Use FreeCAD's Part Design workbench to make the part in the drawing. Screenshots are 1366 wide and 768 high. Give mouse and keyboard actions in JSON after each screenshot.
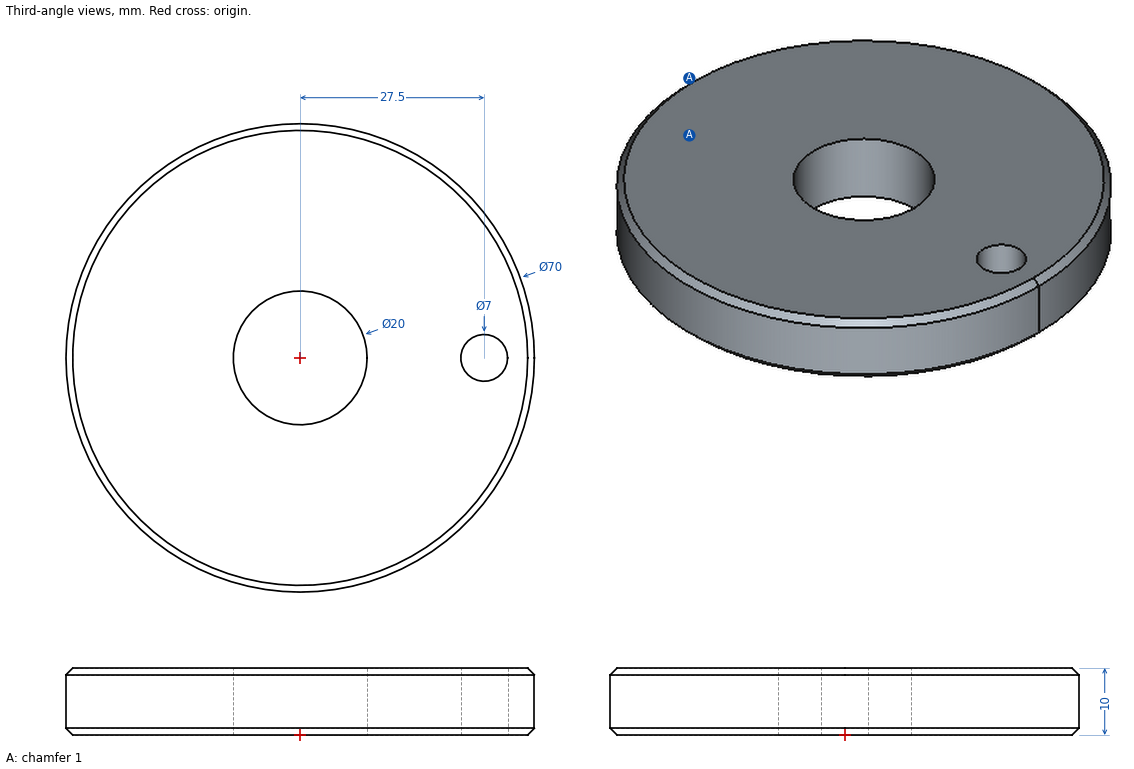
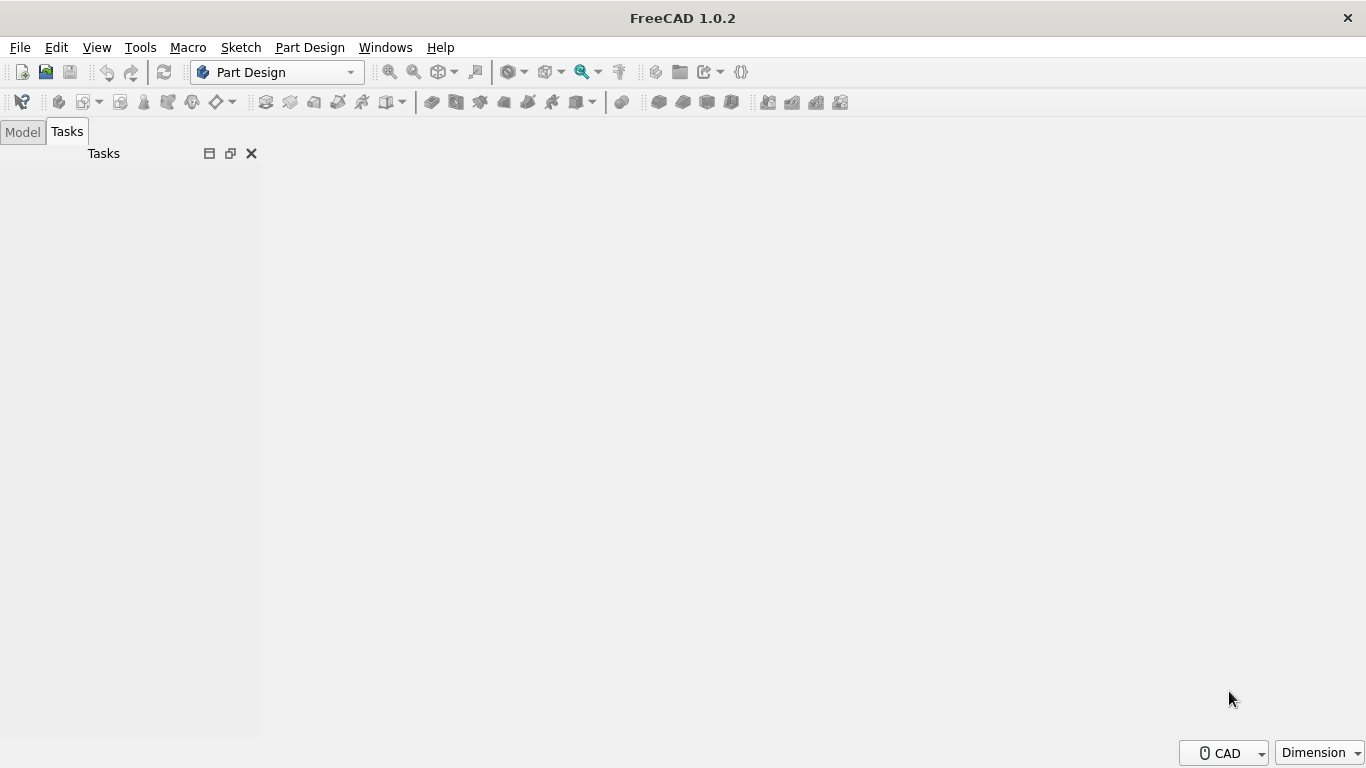
{"action": "left_click", "coordinate": [22, 72]}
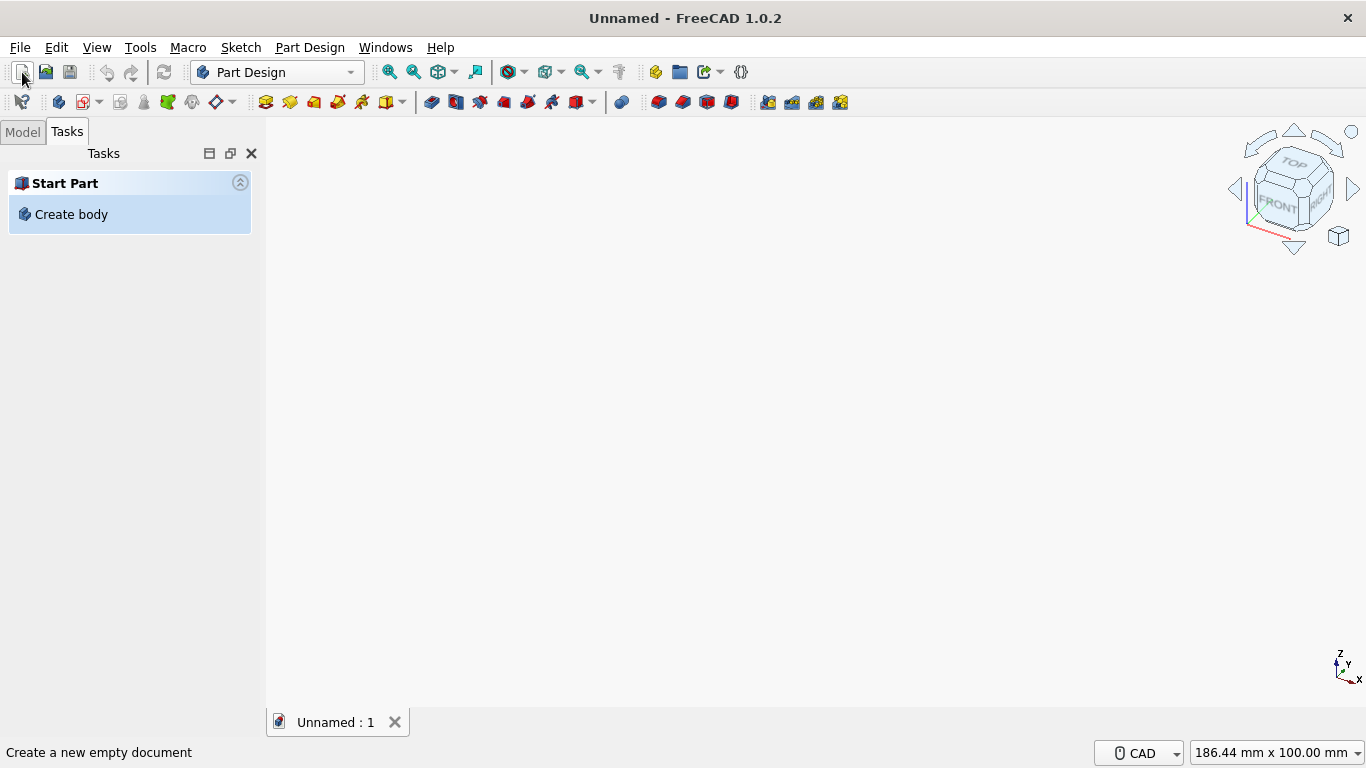
{"action": "left_click", "coordinate": [84, 102]}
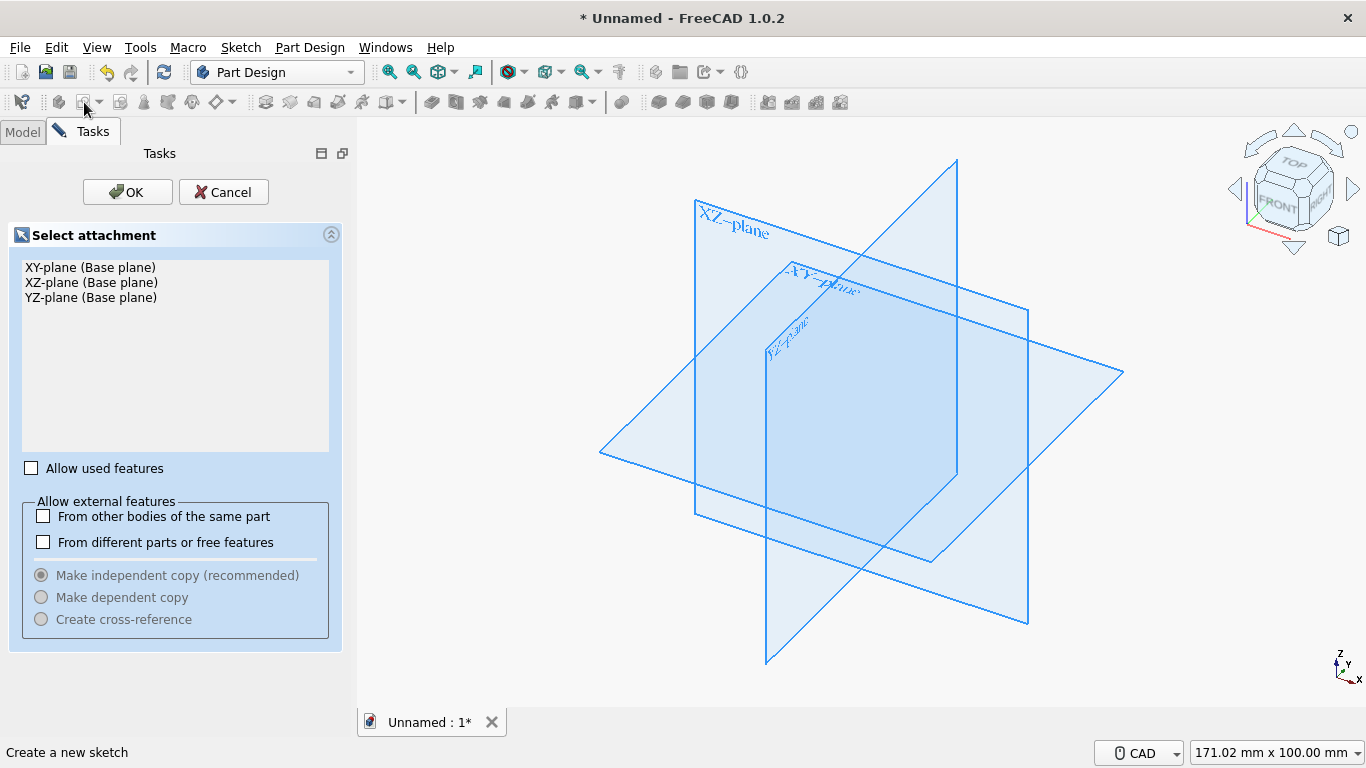
{"action": "left_click", "coordinate": [82, 268]}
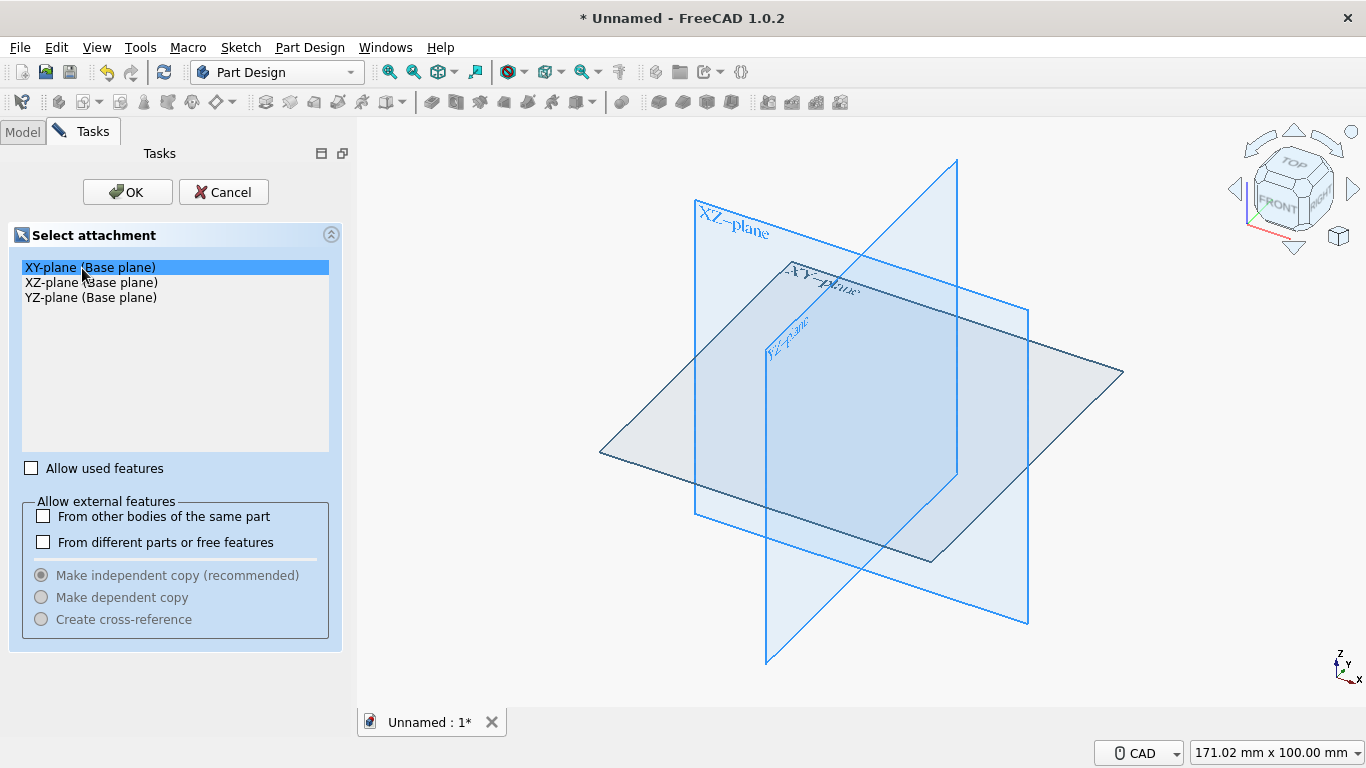
{"action": "left_click", "coordinate": [128, 192]}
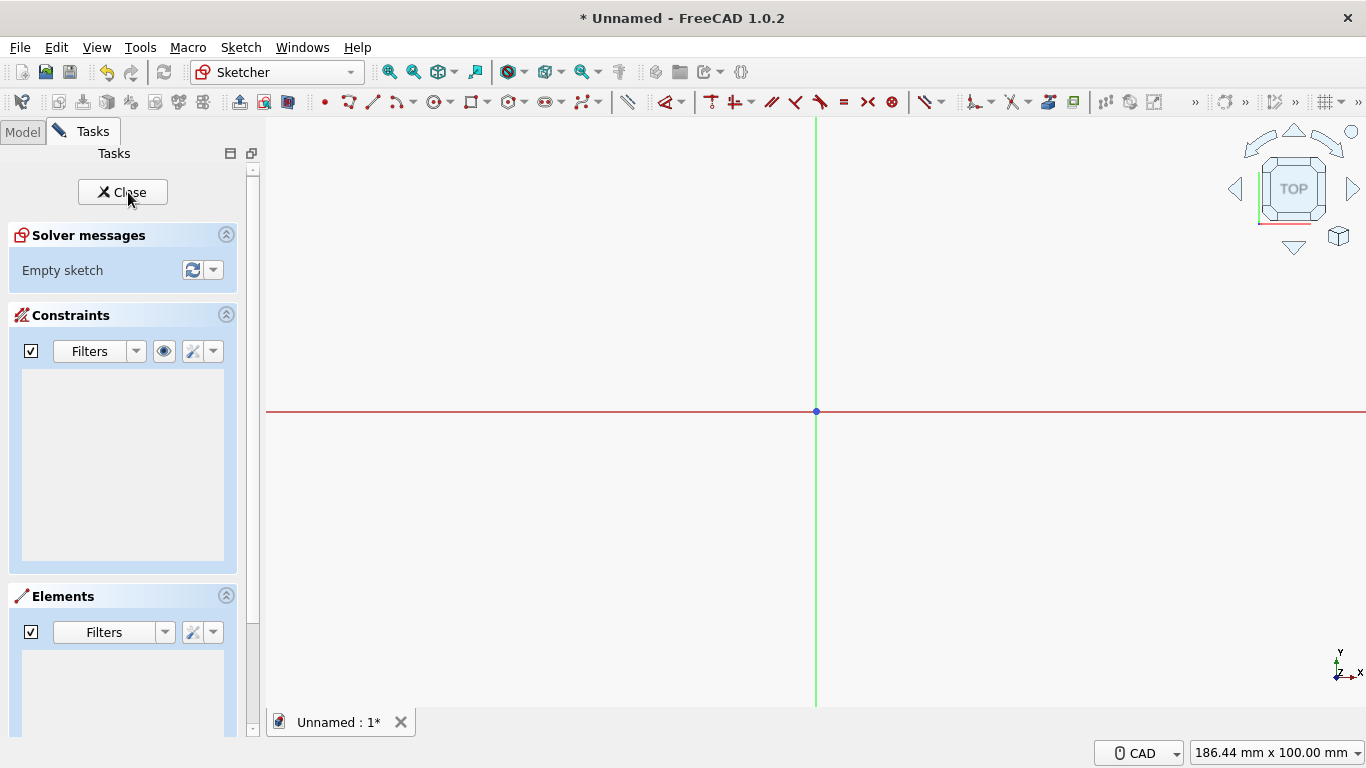
{"action": "left_click", "coordinate": [434, 102]}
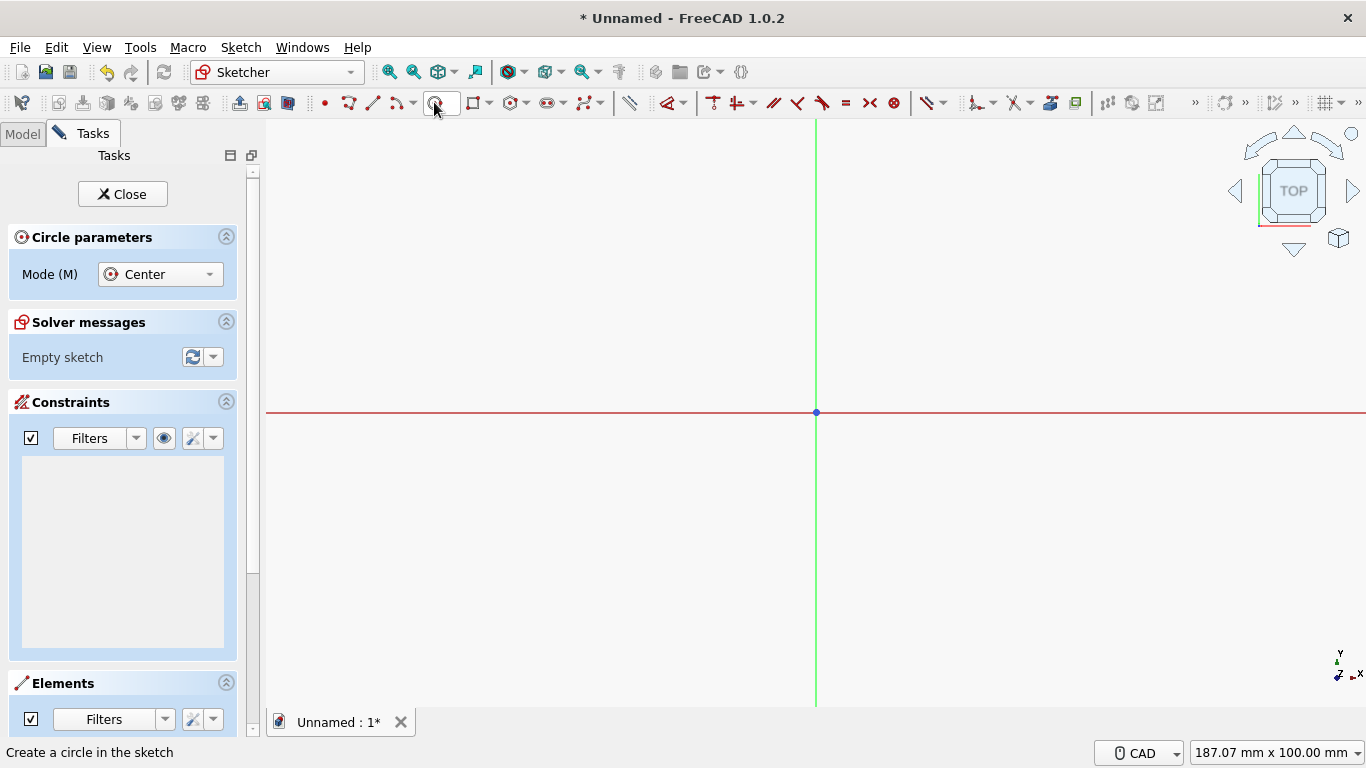
{"action": "left_click", "coordinate": [816, 413]}
{"action": "mouse_move", "coordinate": [962, 267]}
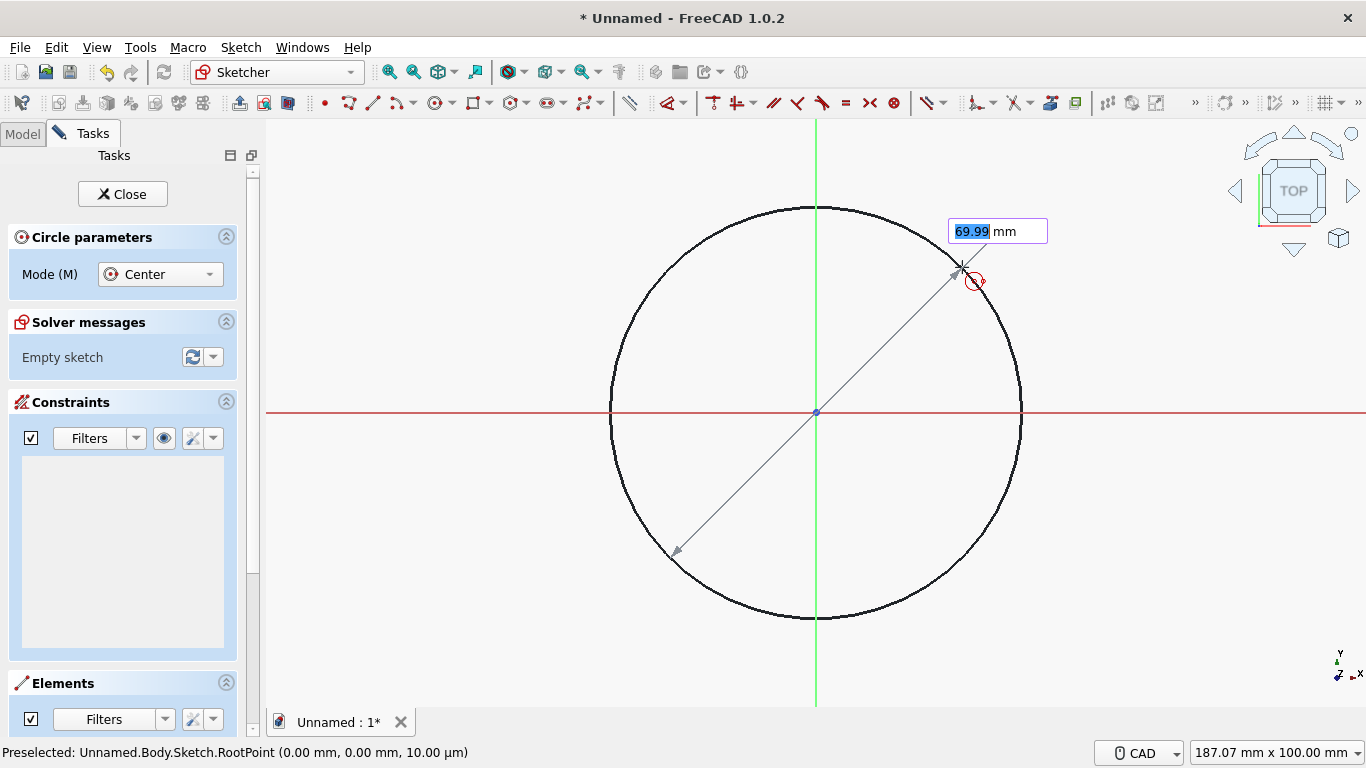
{"action": "type", "text": "70"}
{"action": "key", "text": "Return"}
{"action": "key", "text": "Escape"}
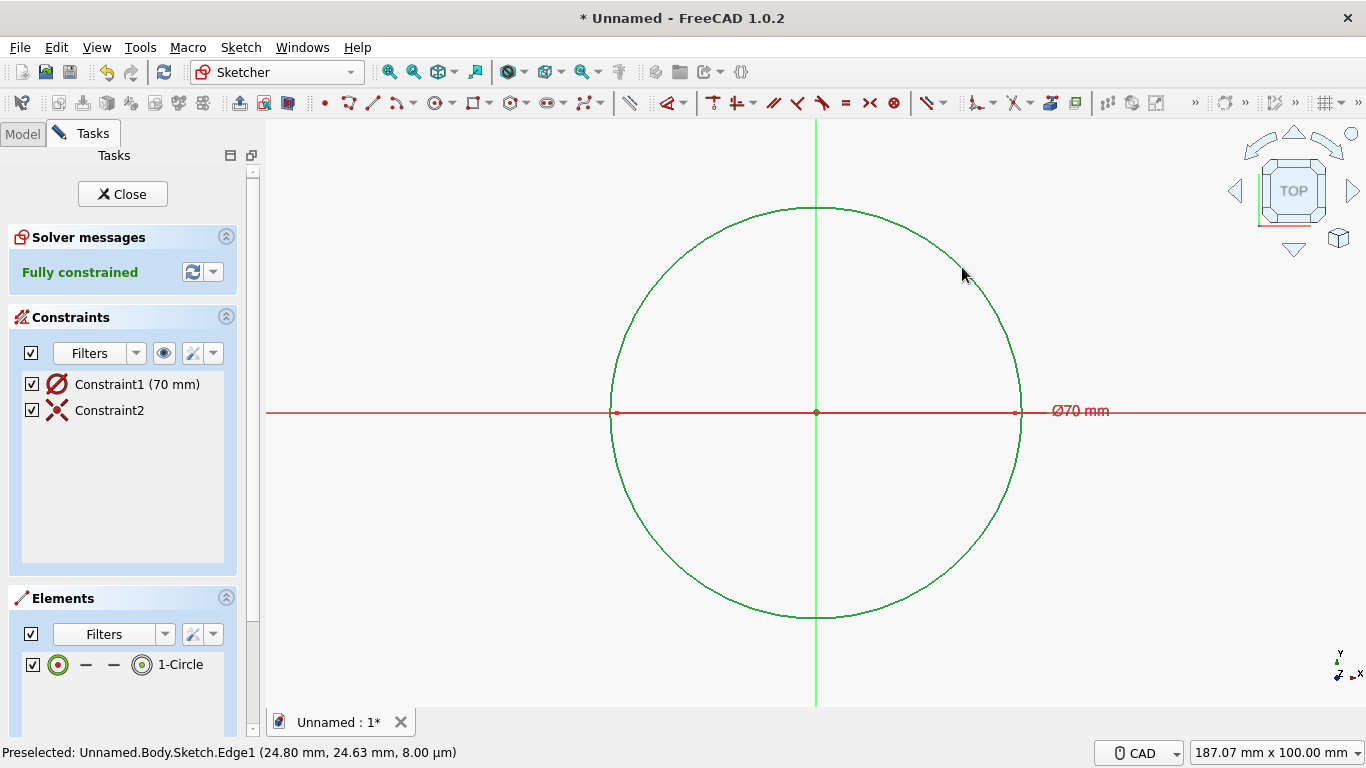
{"action": "left_click", "coordinate": [123, 194]}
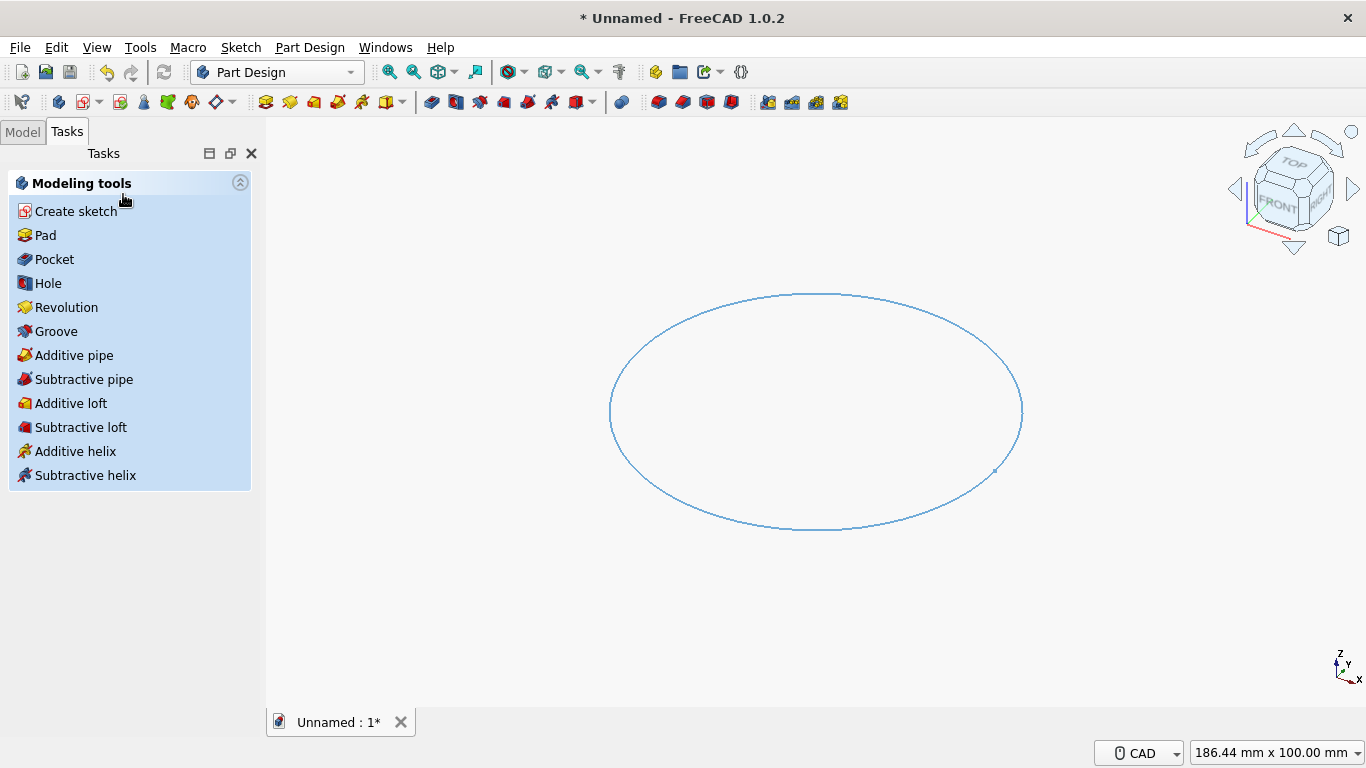
{"action": "left_click", "coordinate": [266, 102]}